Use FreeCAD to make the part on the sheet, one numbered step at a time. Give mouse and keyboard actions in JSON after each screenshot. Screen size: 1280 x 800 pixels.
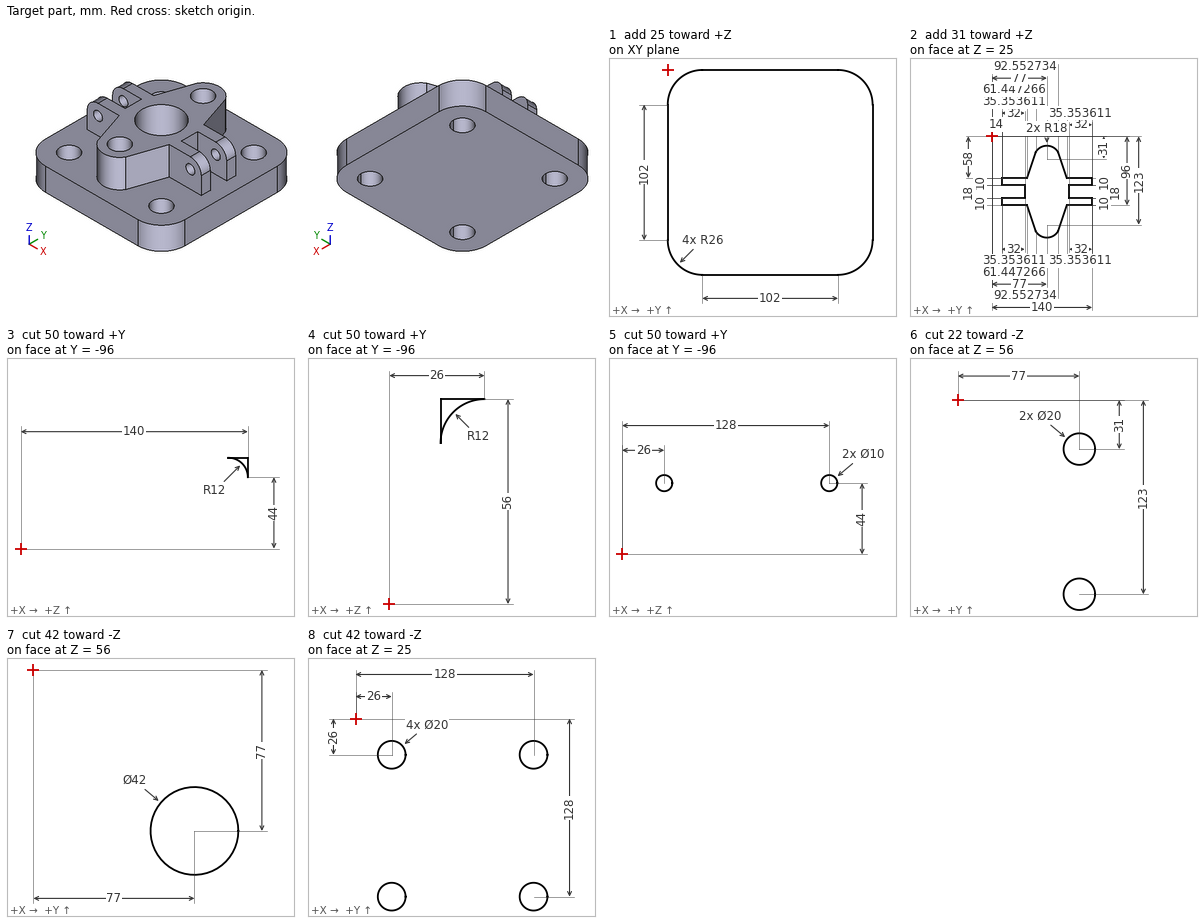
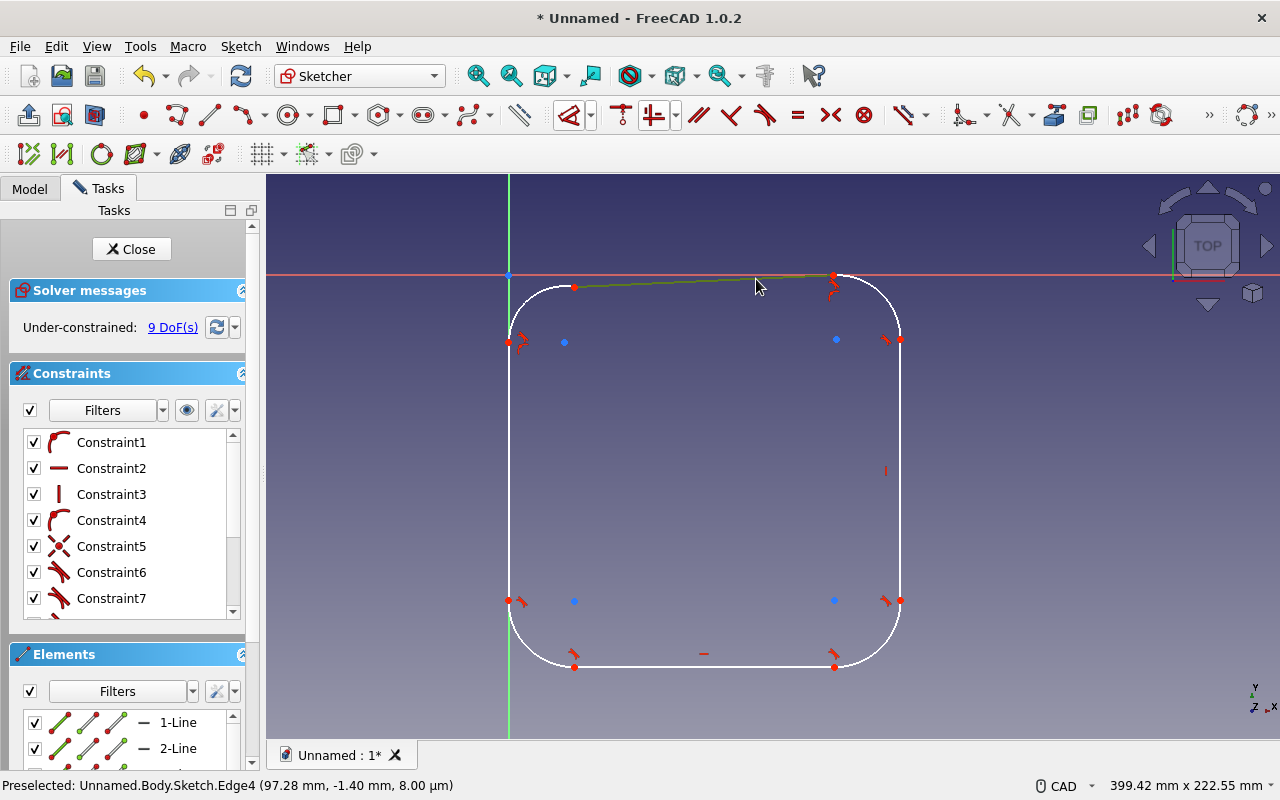
{"action": "left_click", "coordinate": [546, 290]}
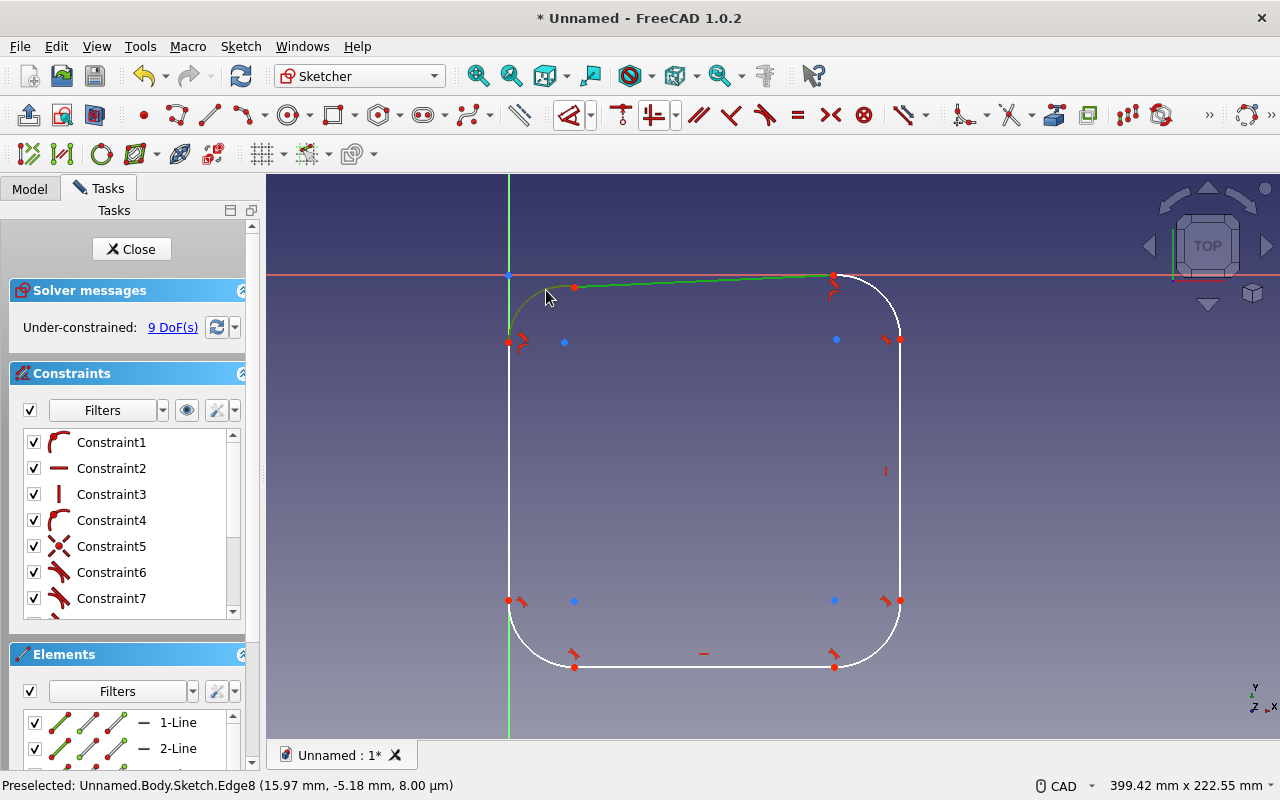
{"action": "left_click", "coordinate": [765, 116]}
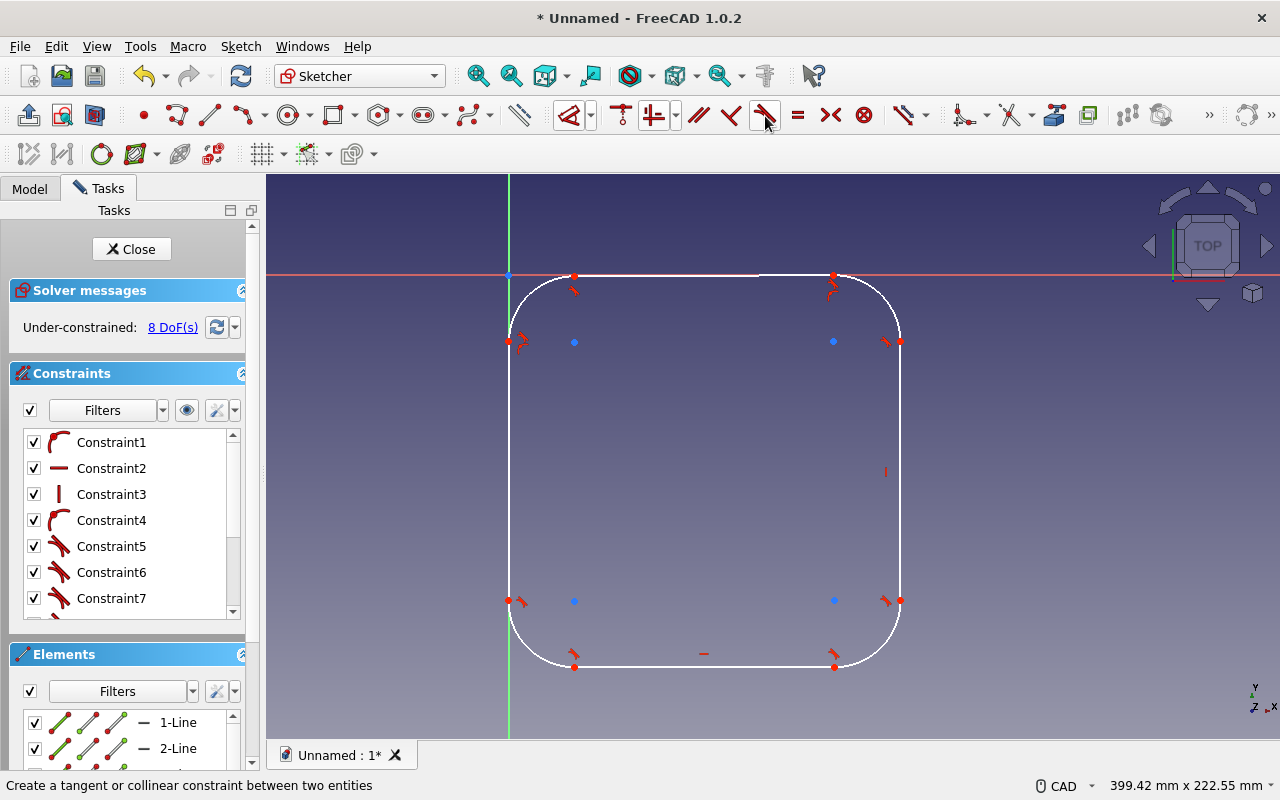
{"action": "left_click", "coordinate": [509, 420]}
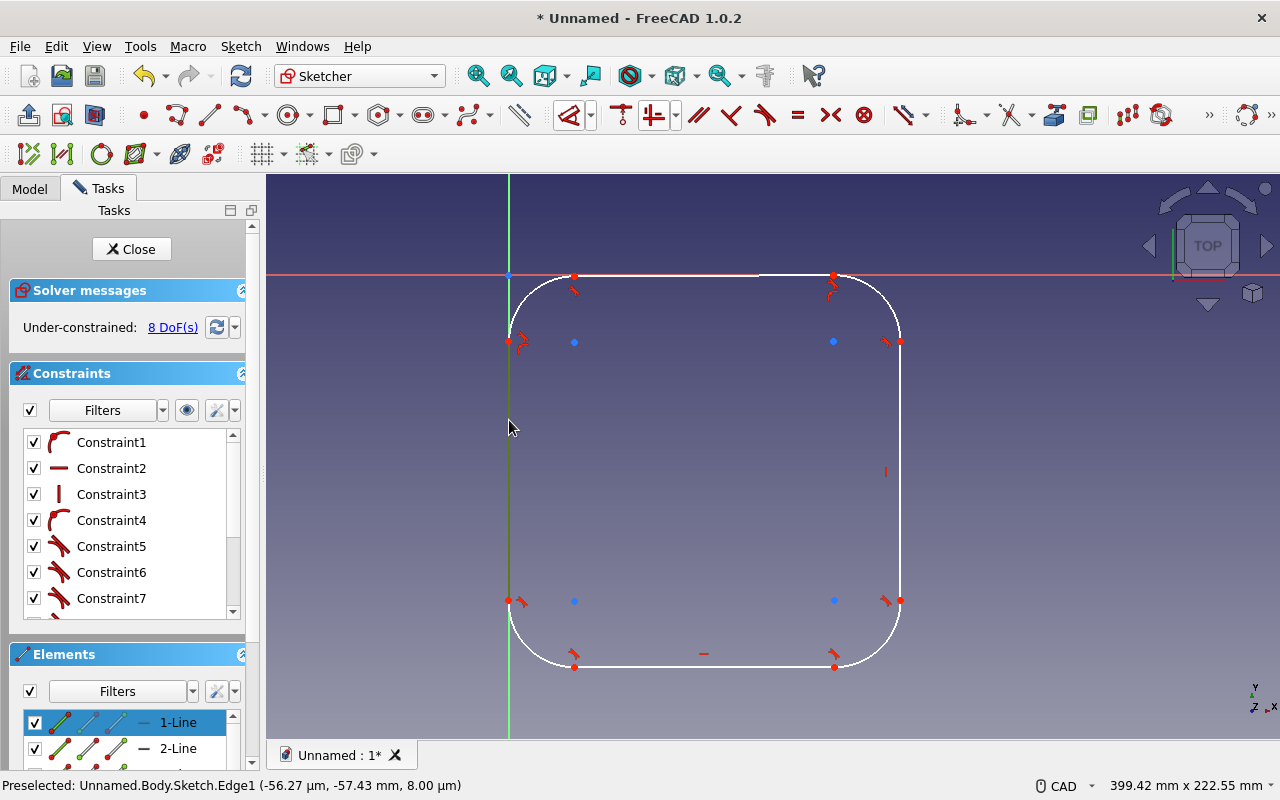
{"action": "left_click", "coordinate": [676, 116]}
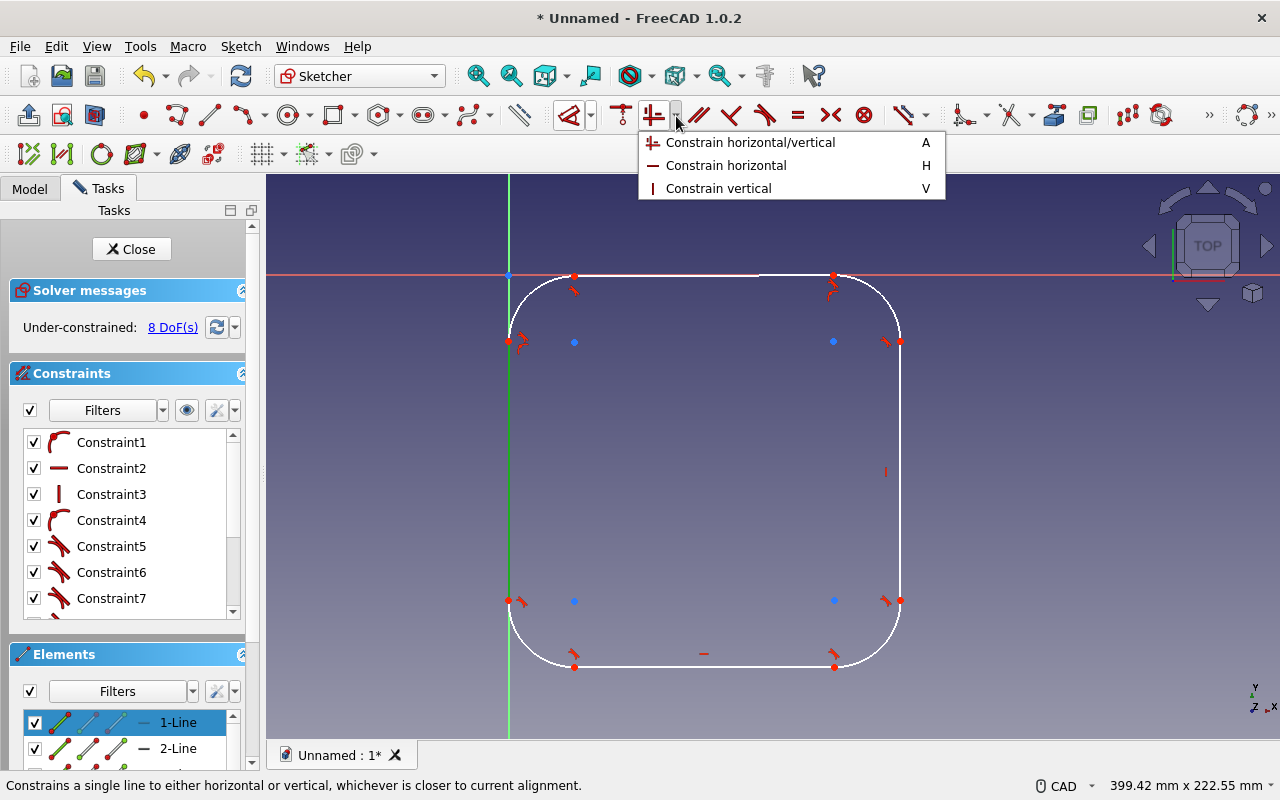
{"action": "left_click", "coordinate": [792, 188]}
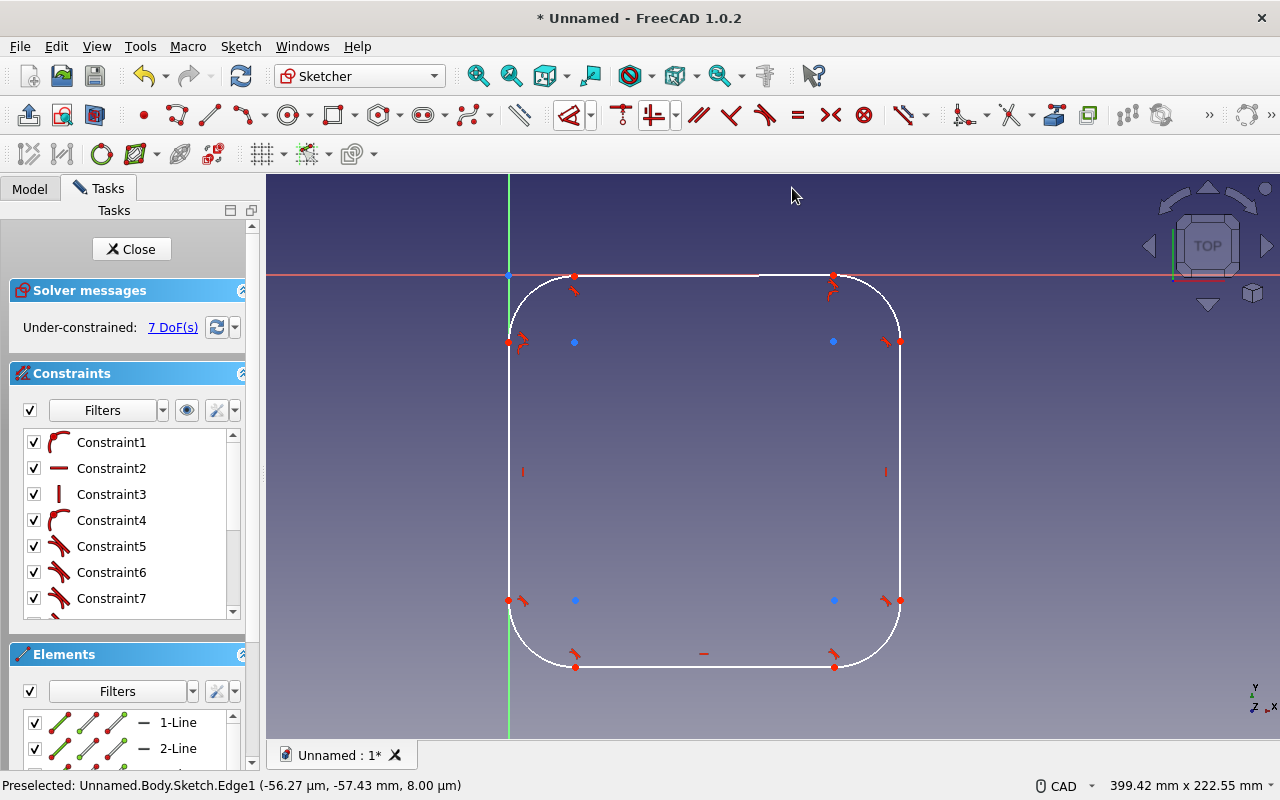
{"action": "left_click", "coordinate": [756, 276]}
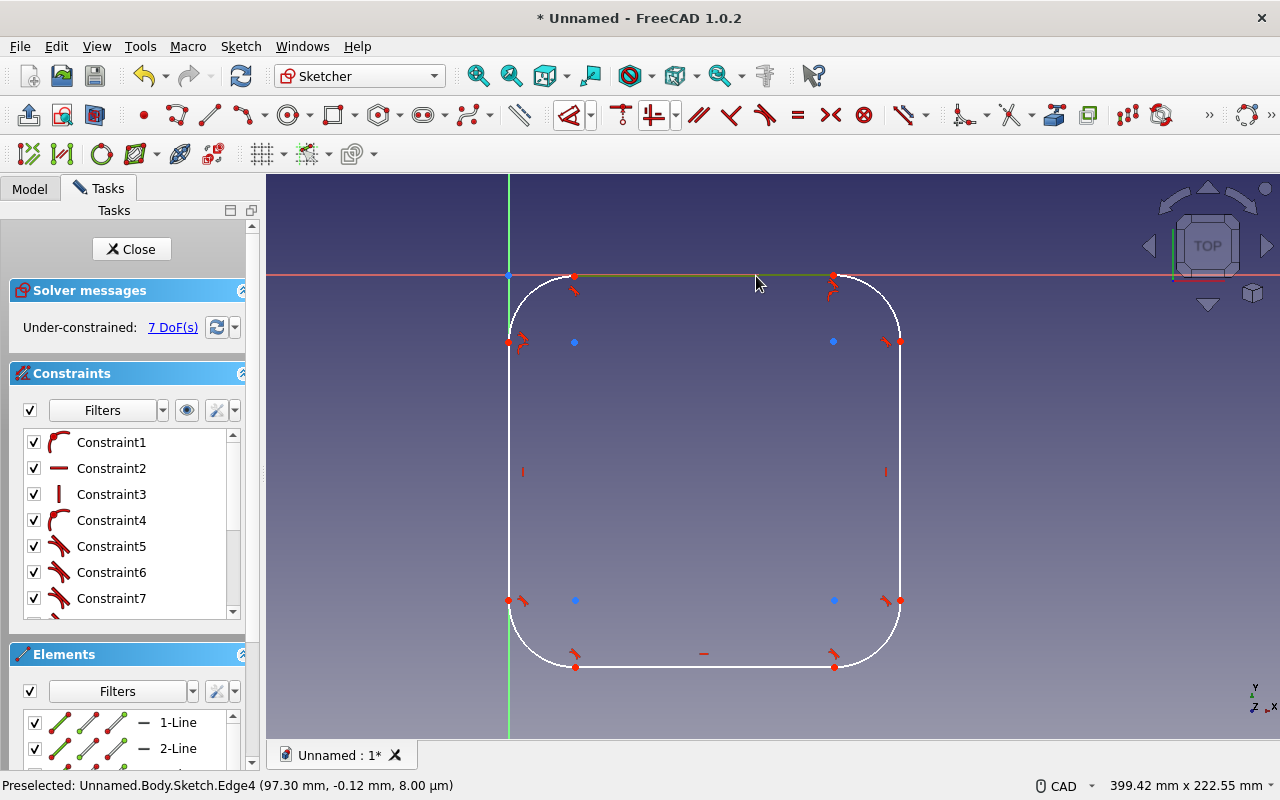
{"action": "left_click", "coordinate": [676, 116]}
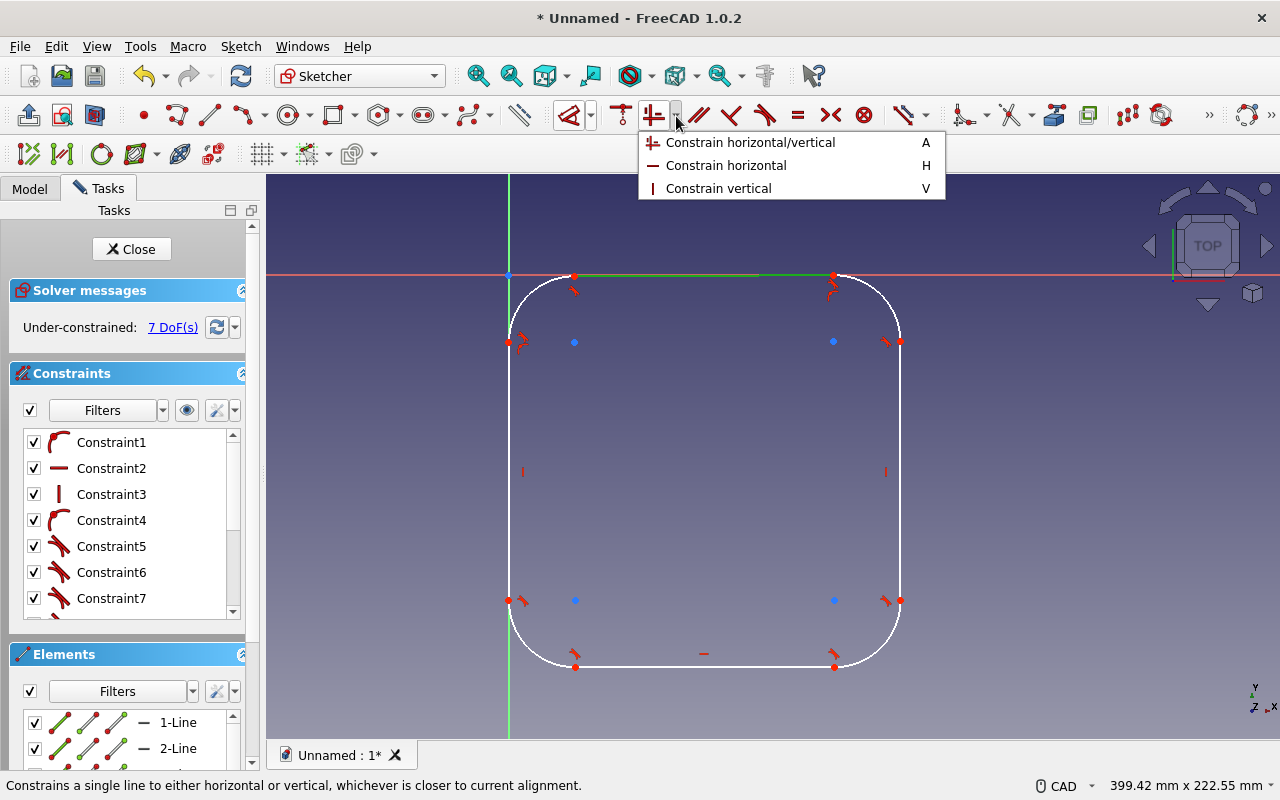
{"action": "left_click", "coordinate": [792, 166]}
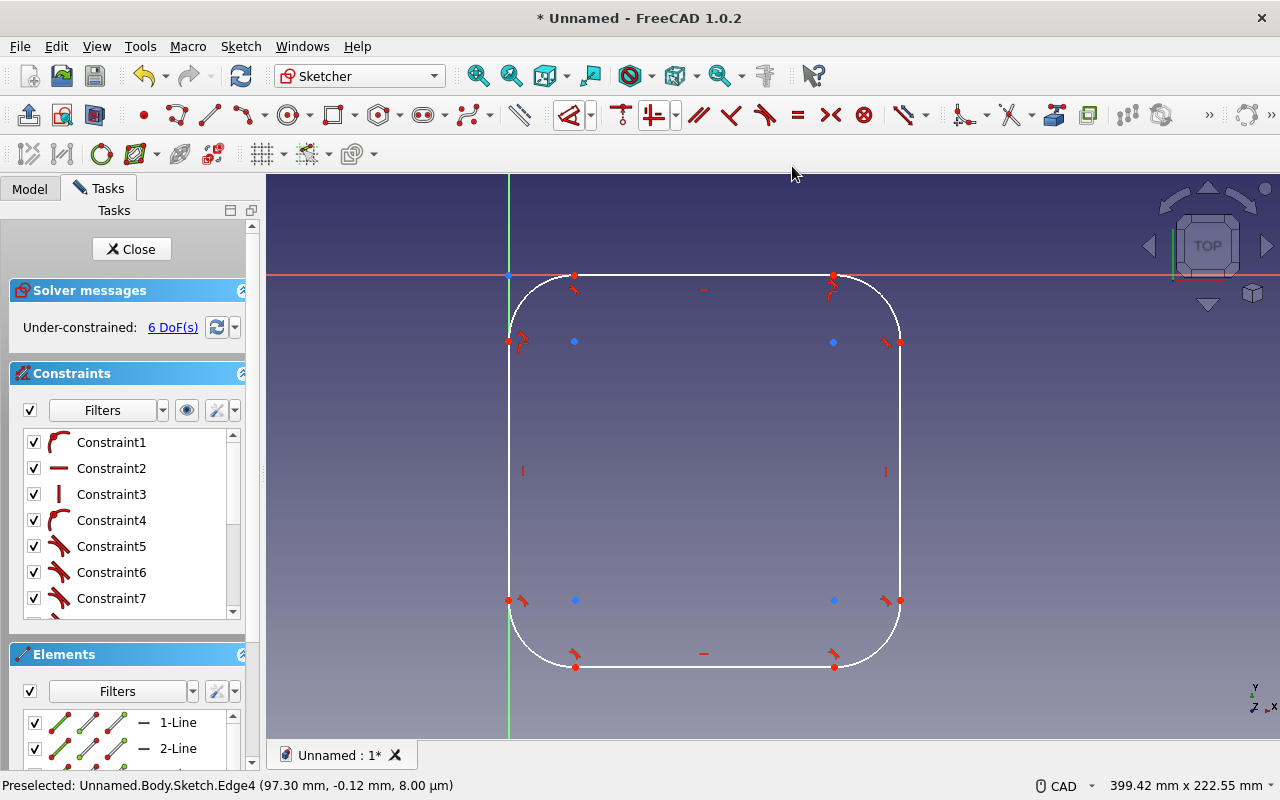
{"action": "left_click", "coordinate": [545, 660]}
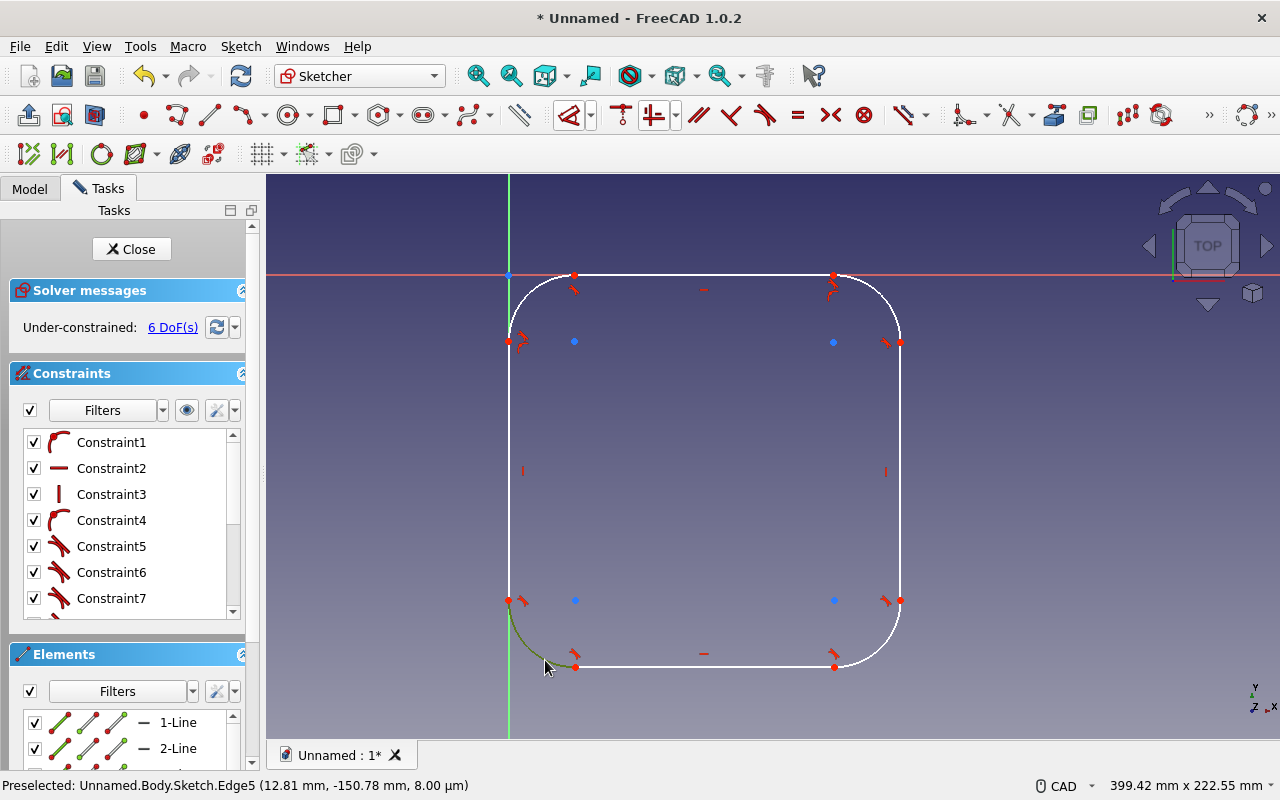
{"action": "left_click", "coordinate": [864, 660]}